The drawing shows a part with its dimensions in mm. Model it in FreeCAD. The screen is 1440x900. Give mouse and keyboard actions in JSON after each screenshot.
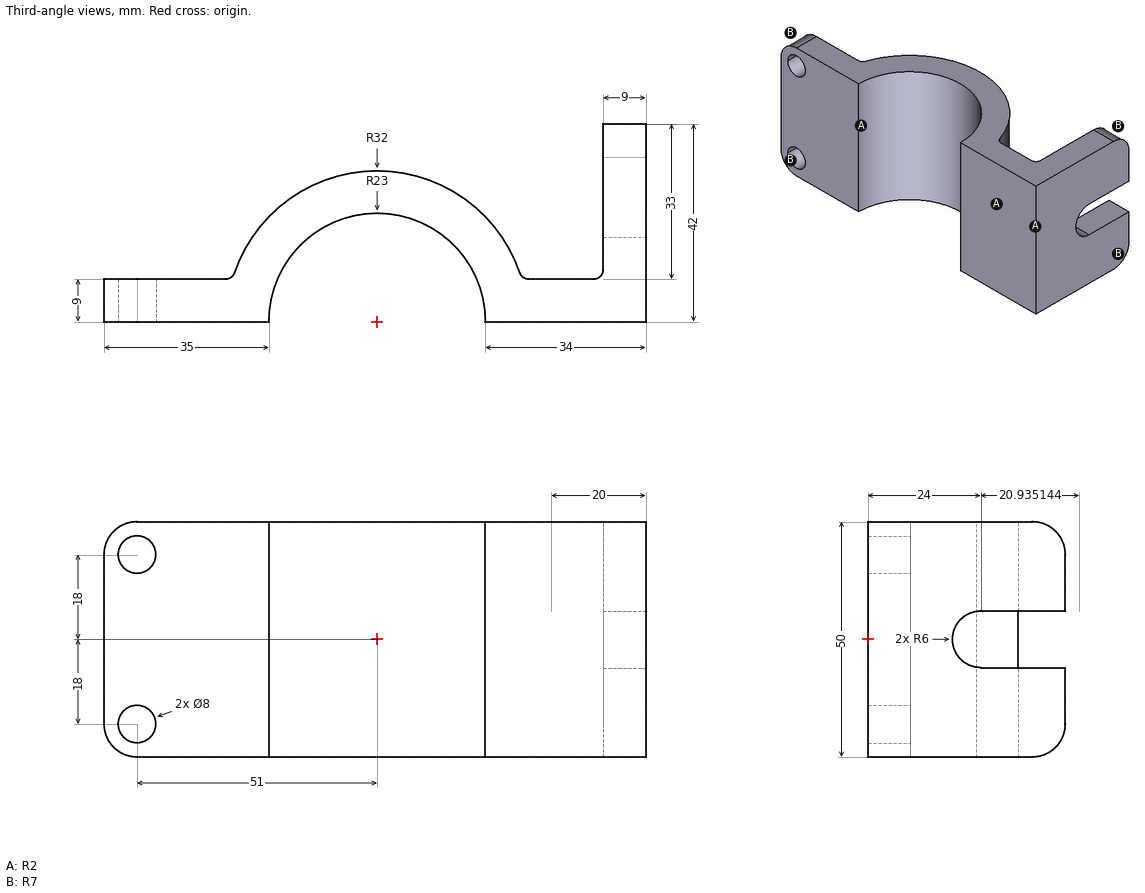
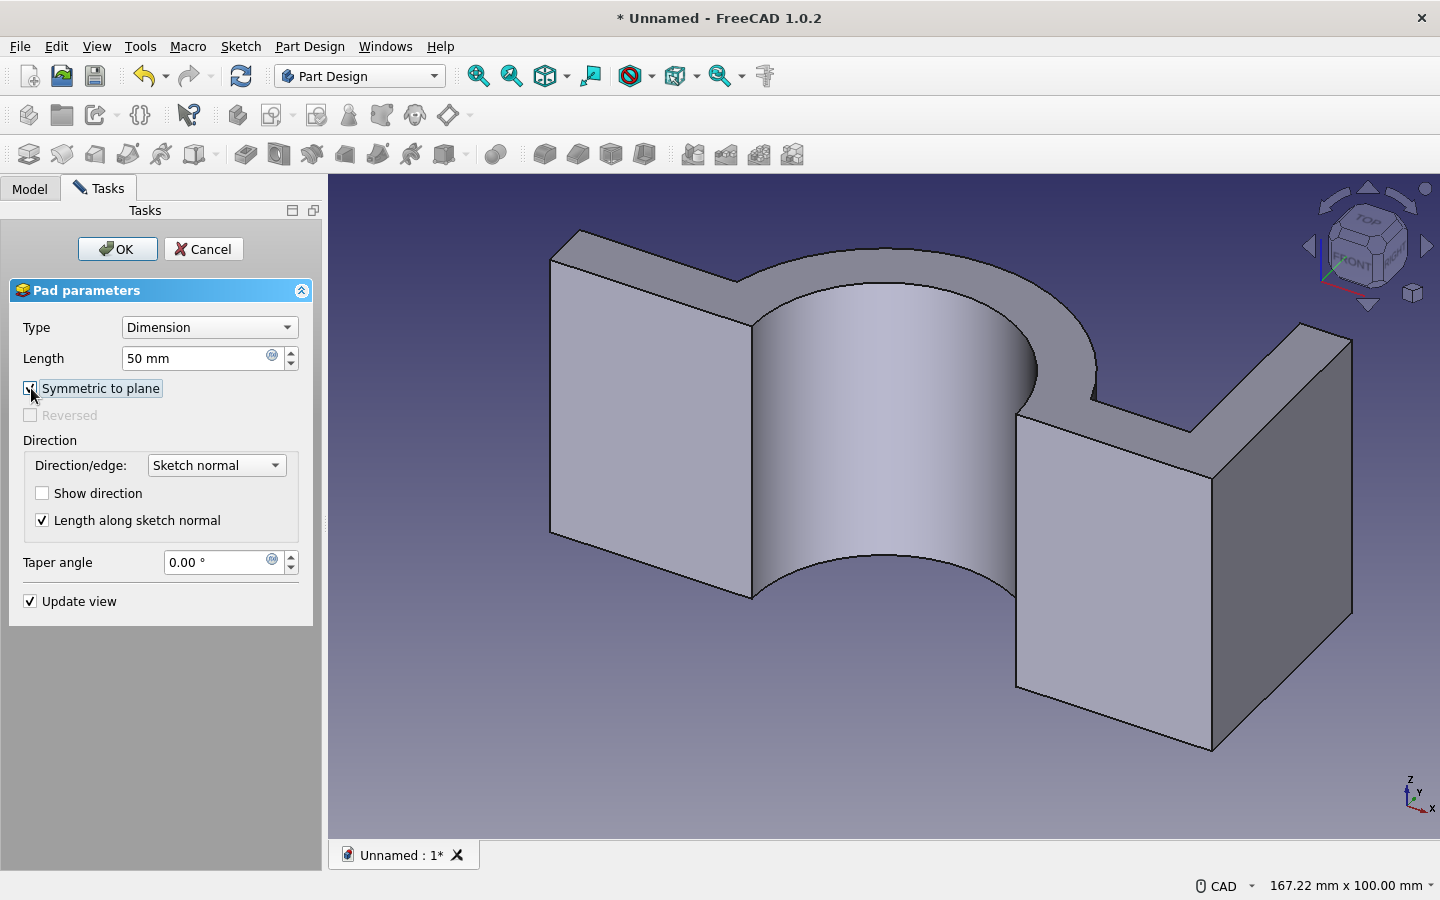
{"action": "left_click", "coordinate": [118, 249]}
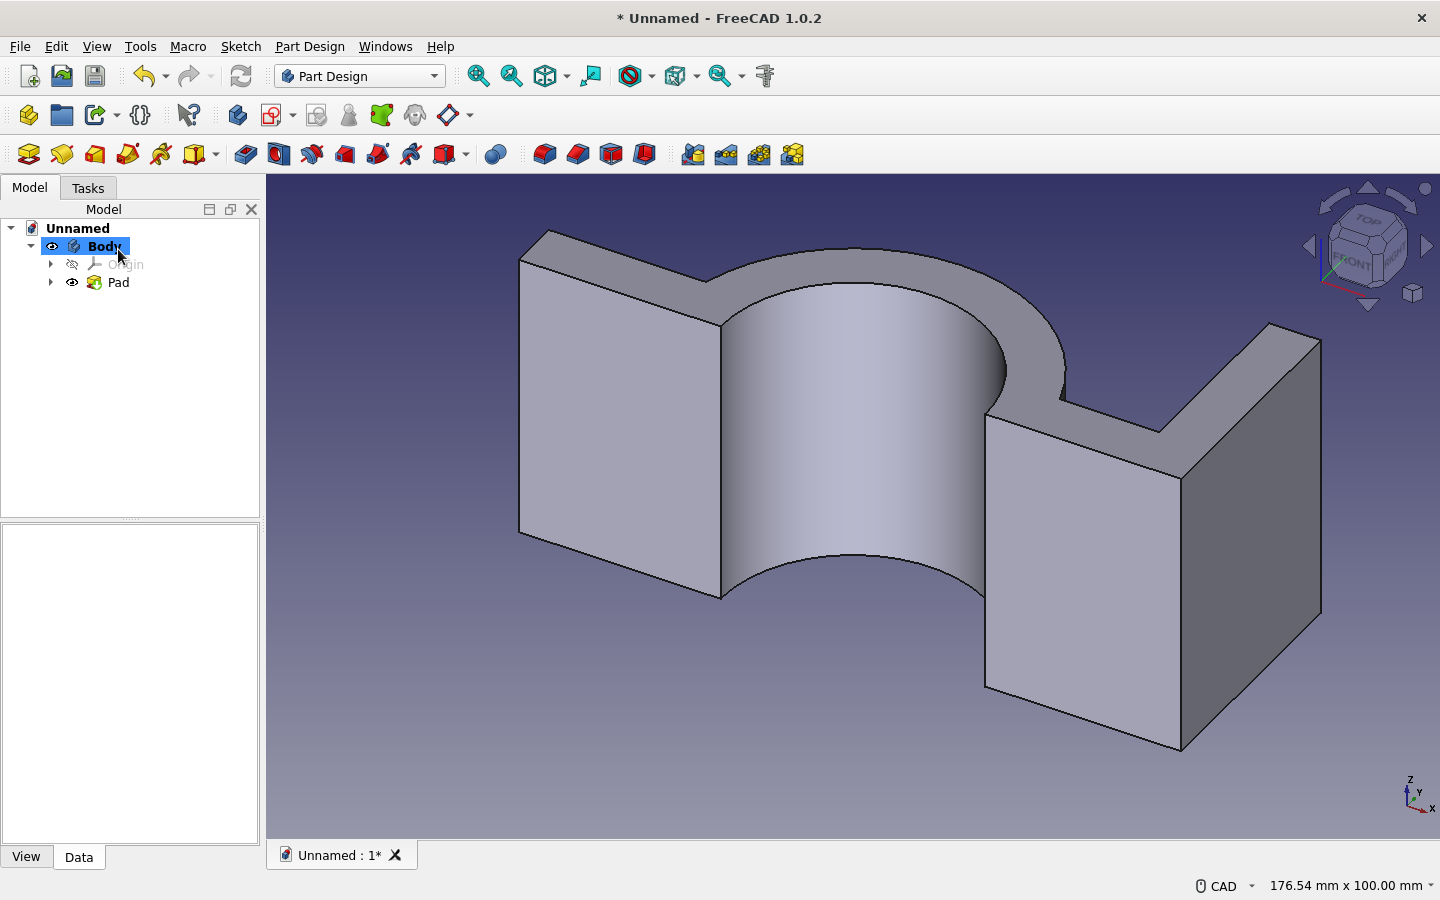
{"action": "left_click", "coordinate": [479, 76]}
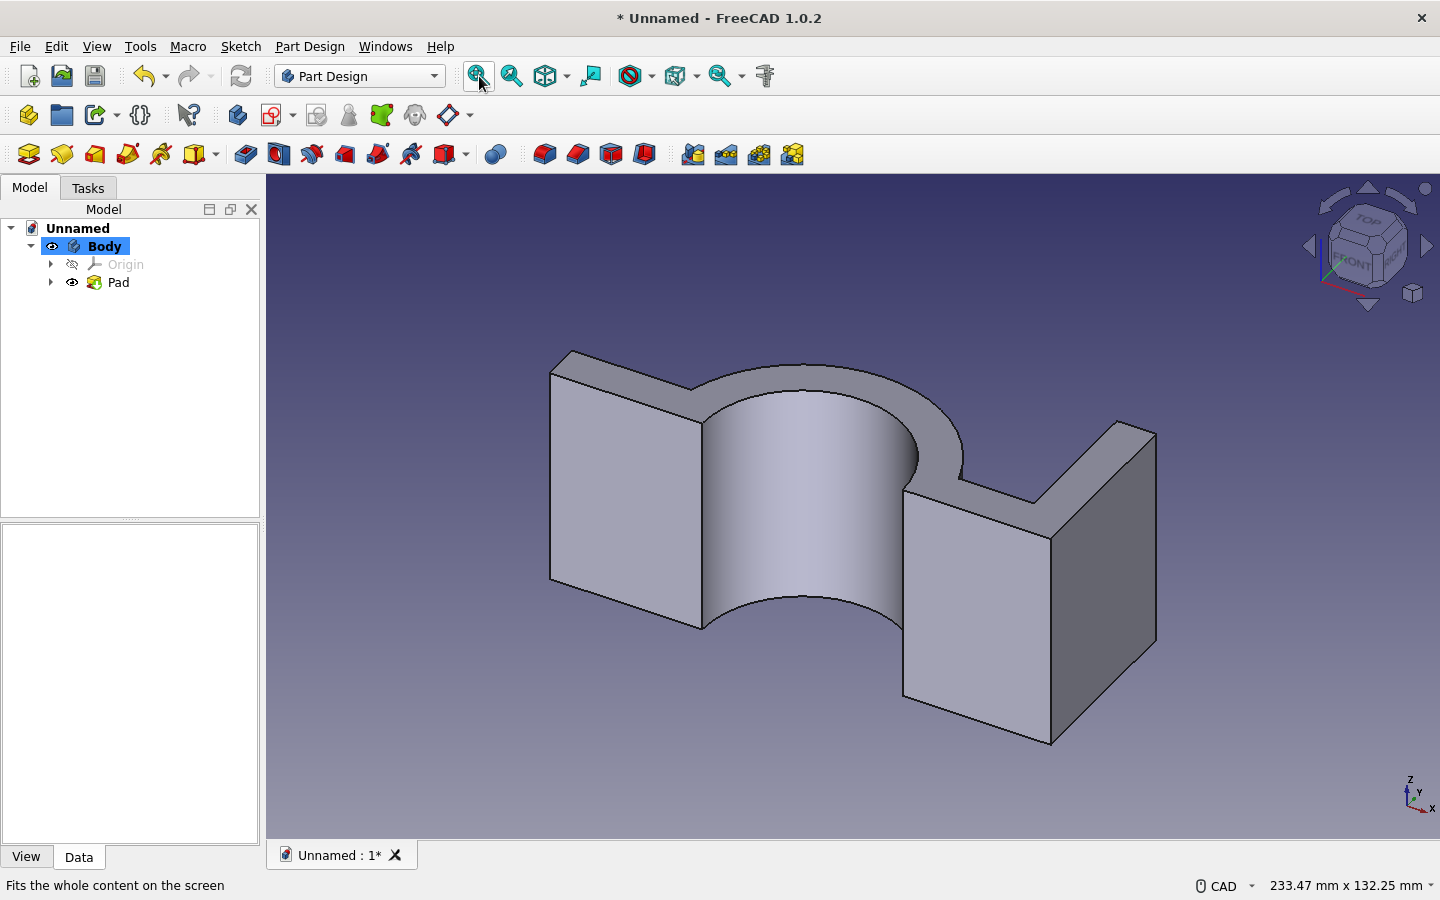
{"action": "key", "text": "0"}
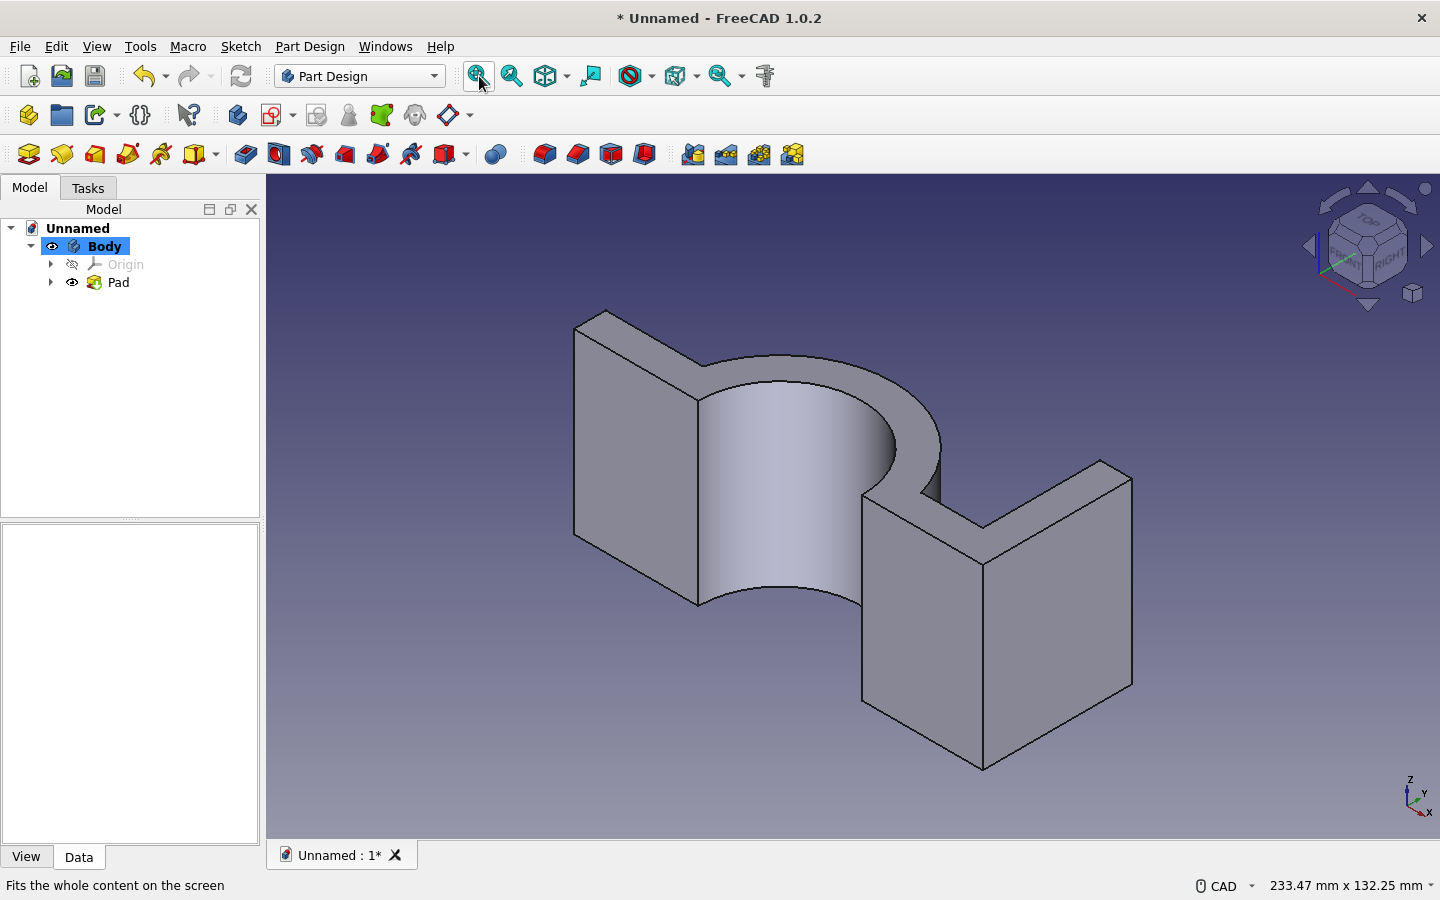
{"action": "key", "text": "2"}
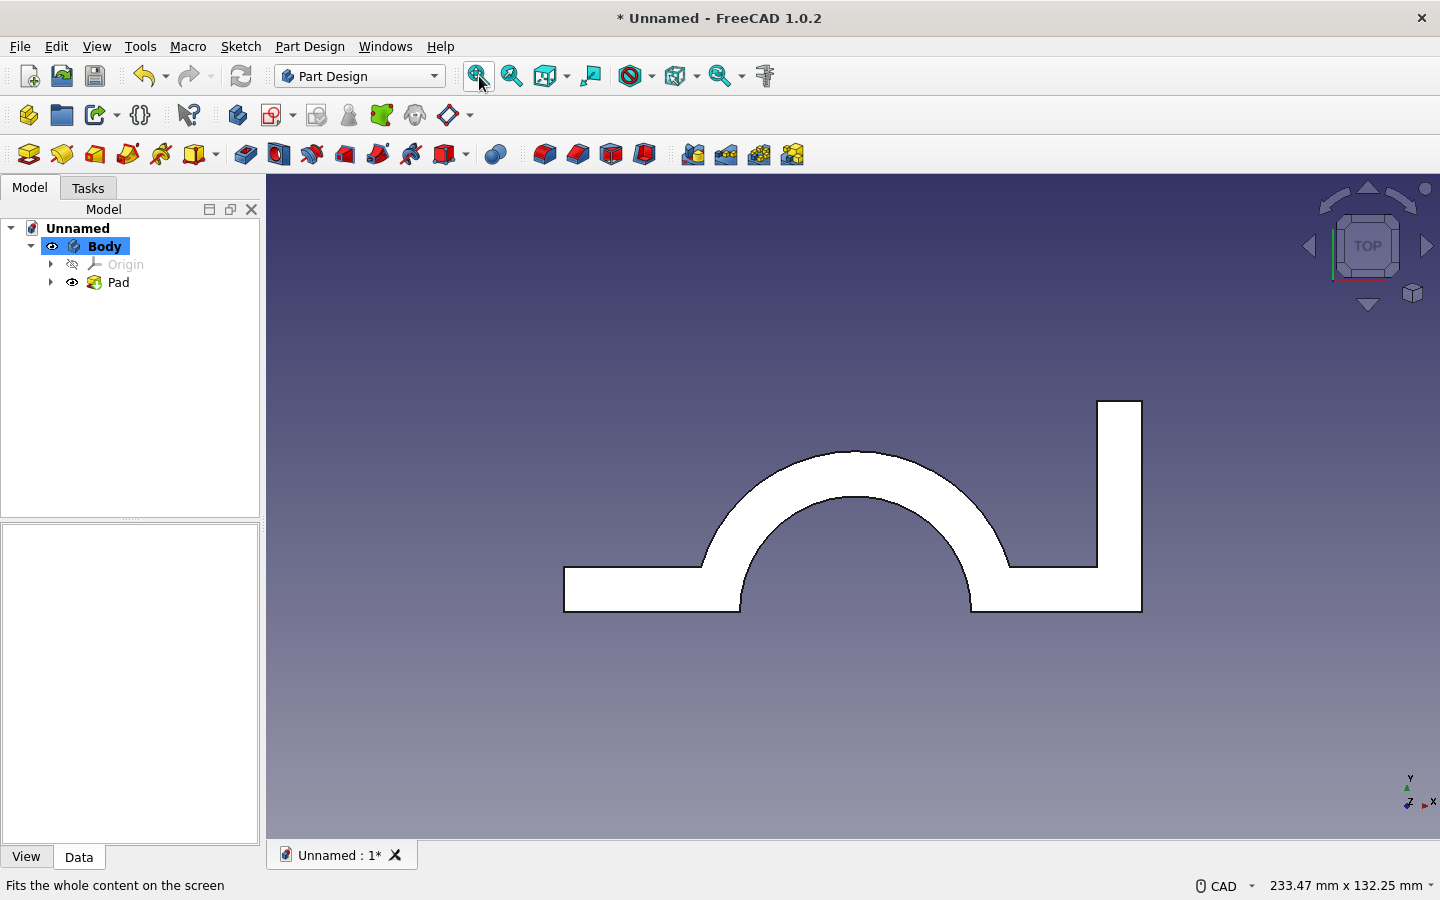
{"action": "key", "text": "1"}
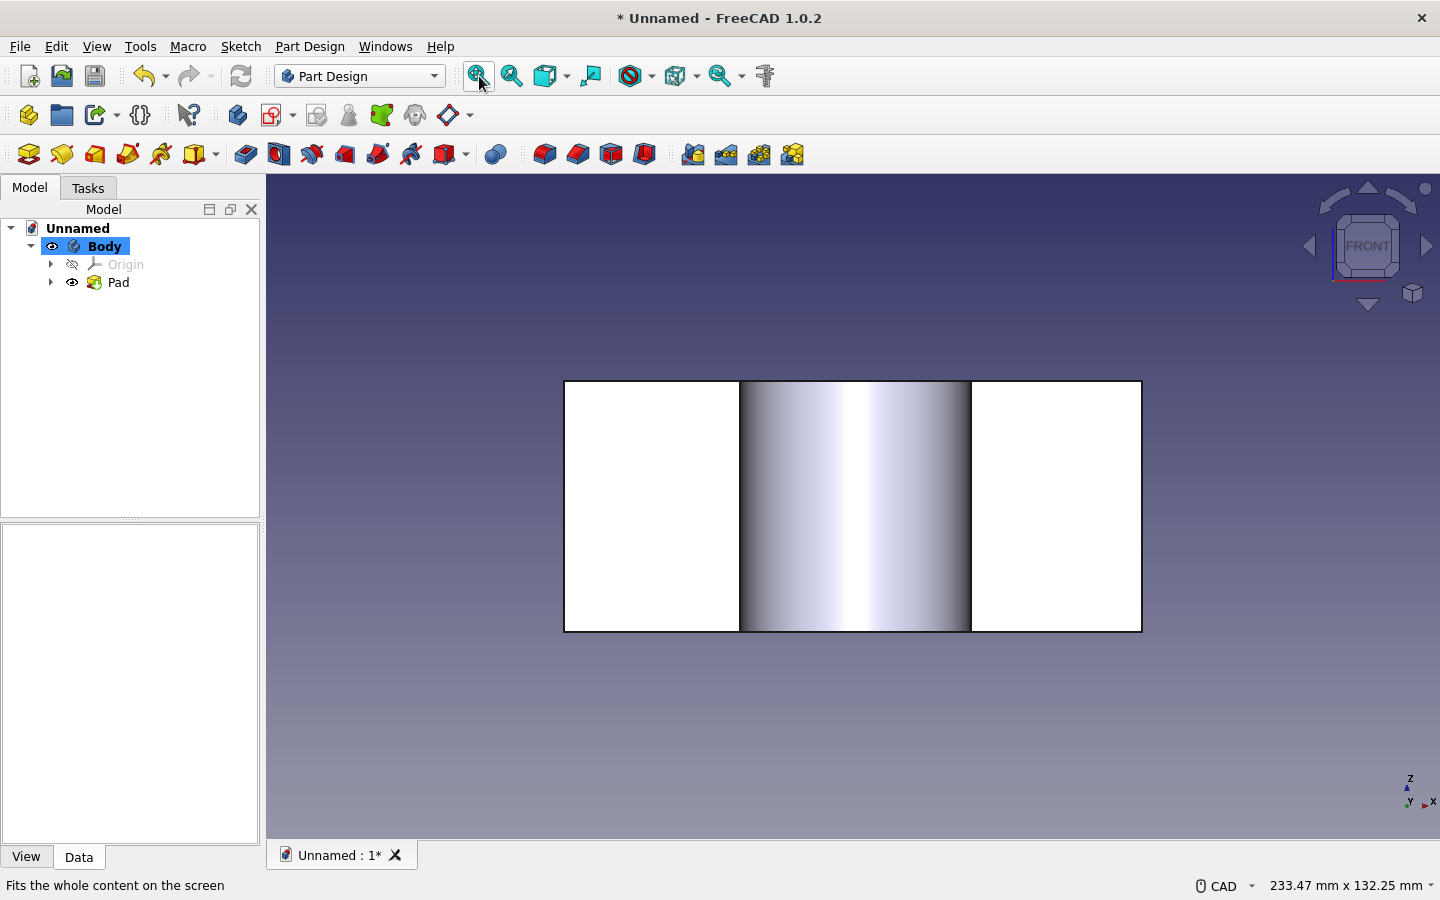
{"action": "key", "text": "3"}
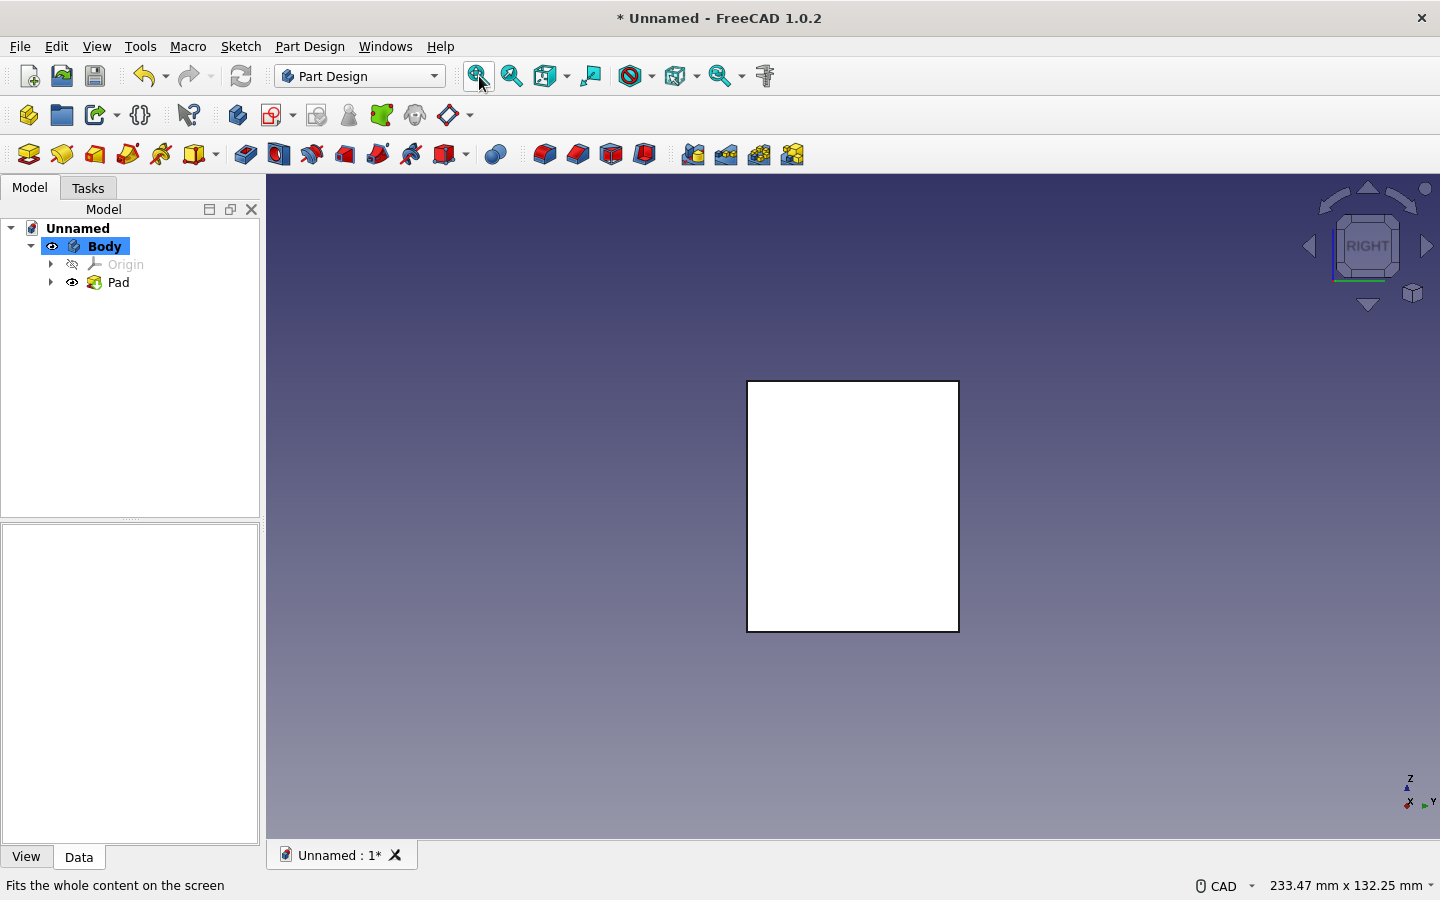
{"action": "left_click", "coordinate": [479, 76]}